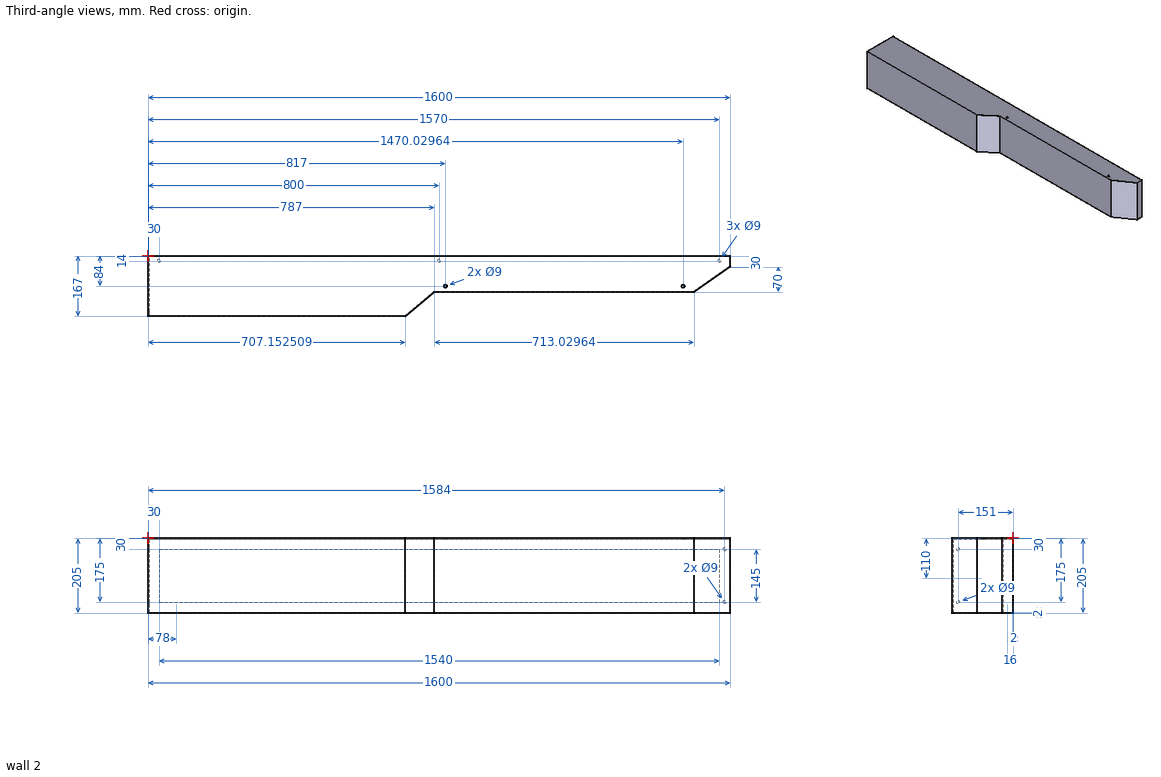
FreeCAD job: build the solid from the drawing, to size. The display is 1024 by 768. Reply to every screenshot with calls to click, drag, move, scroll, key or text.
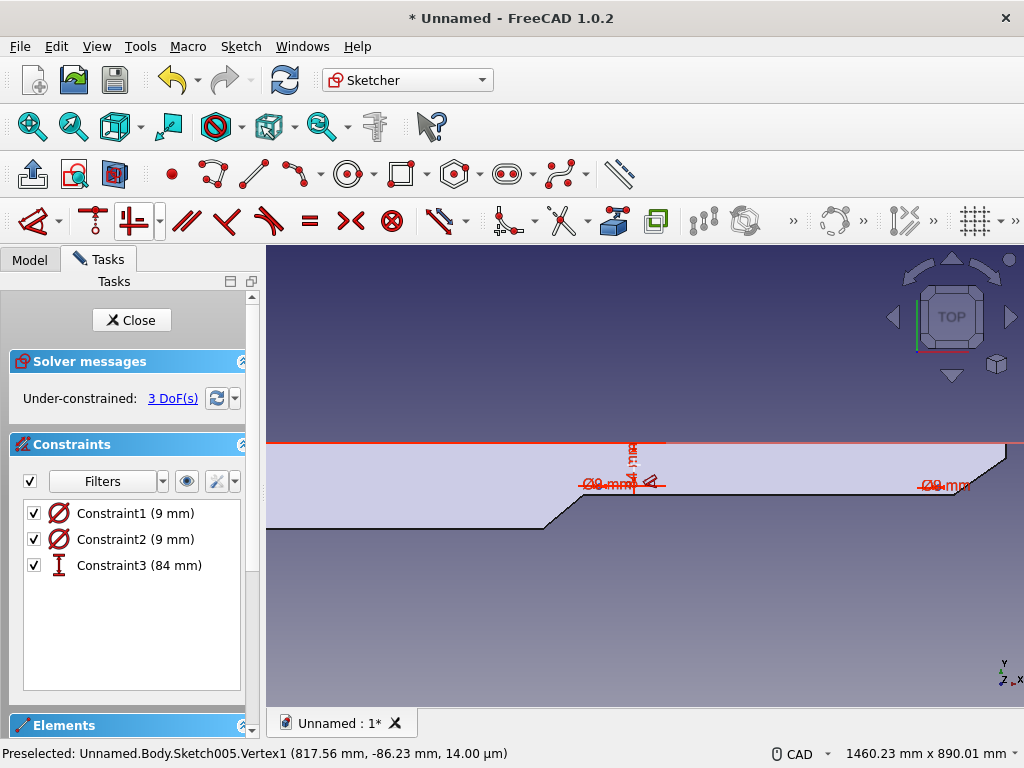
scroll(599, 488, down, 3)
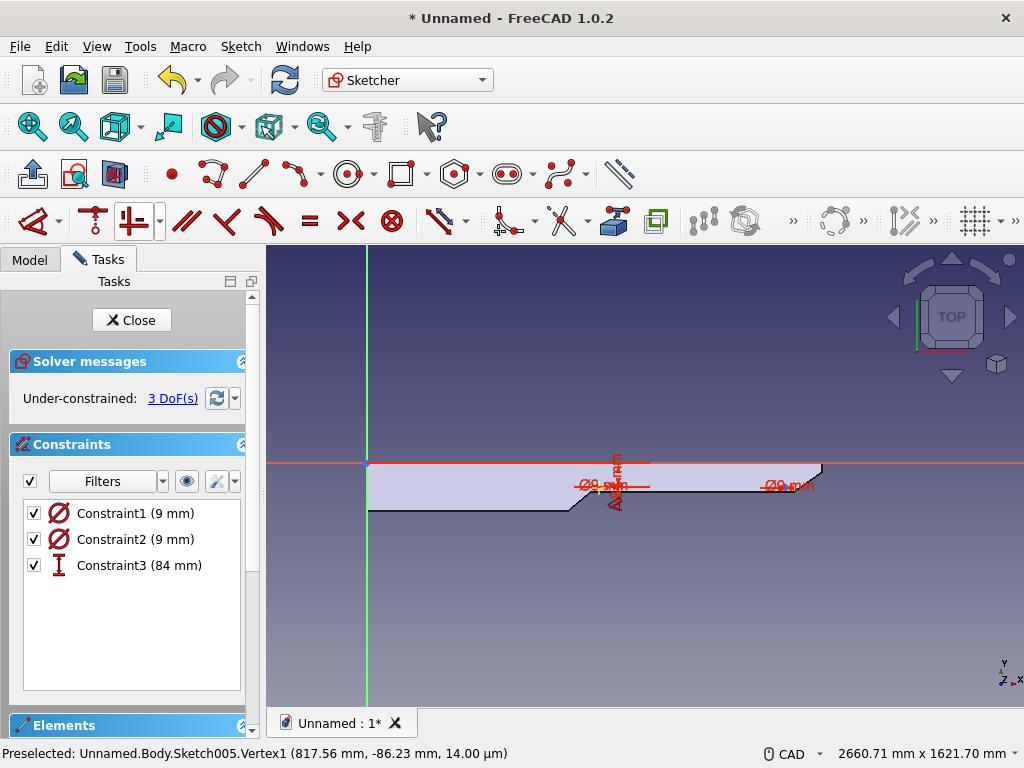
scroll(786, 488, up, 3)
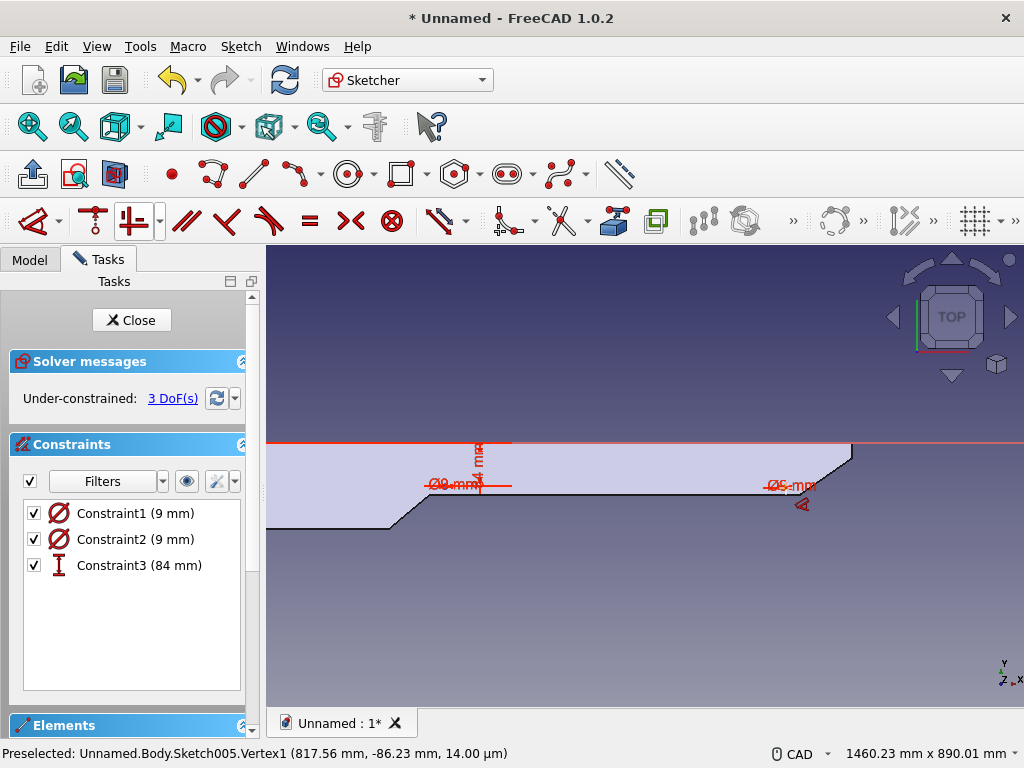
click(785, 488)
click(819, 465)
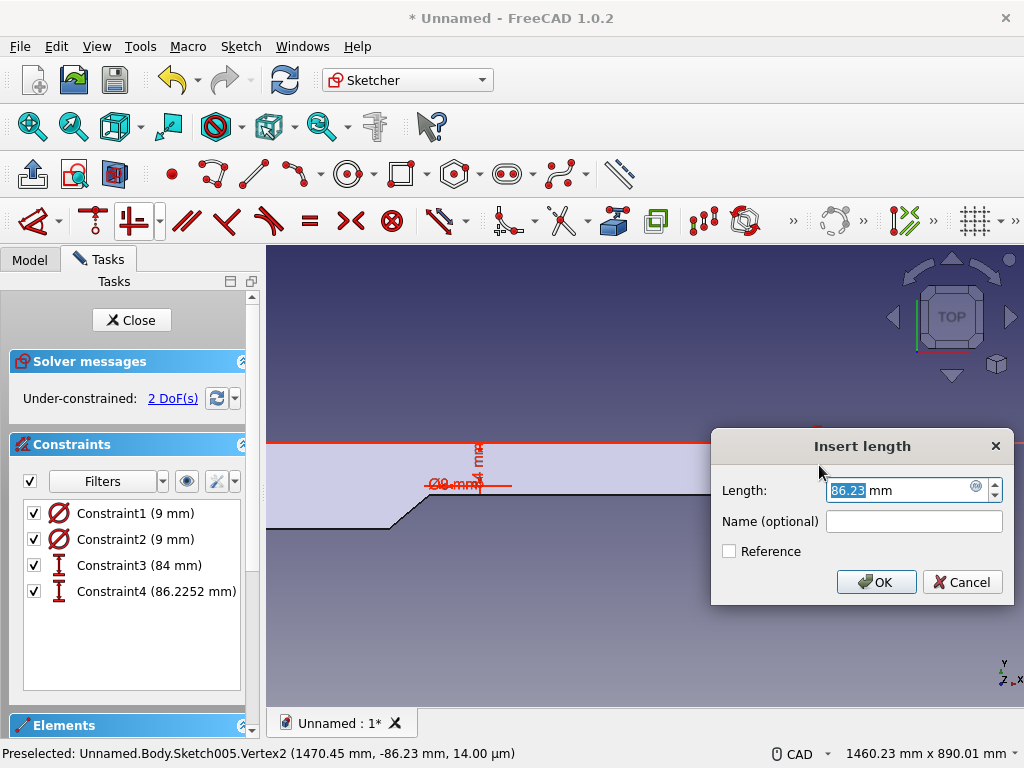
text(84)
key(Return)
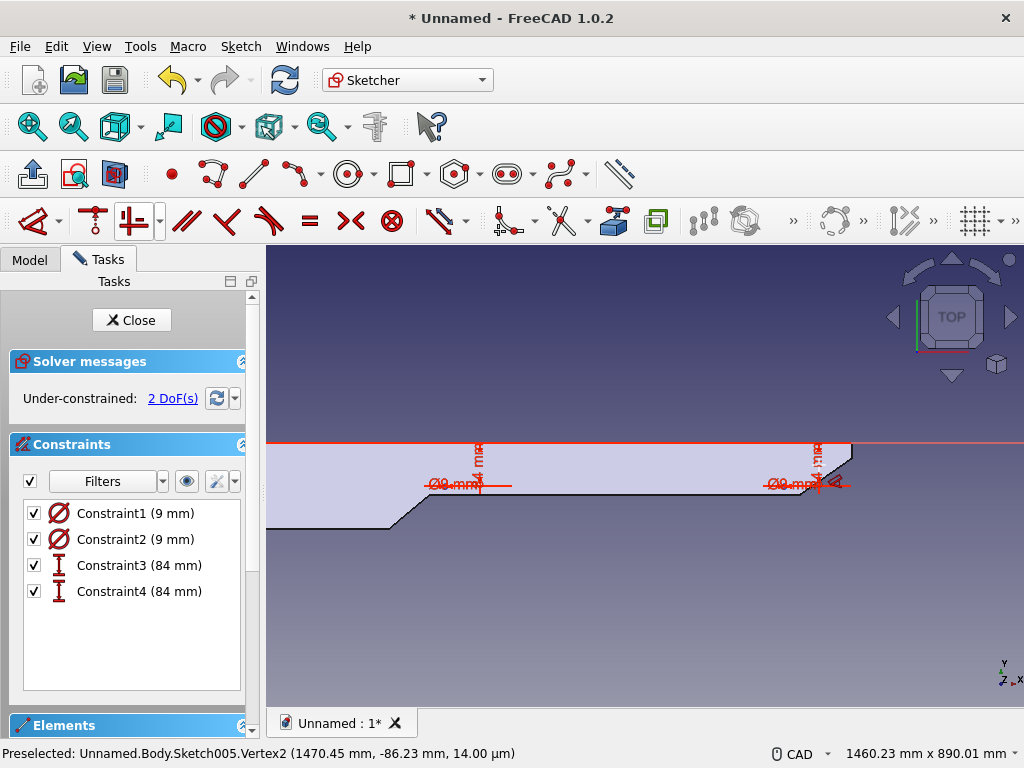
click(446, 486)
click(370, 409)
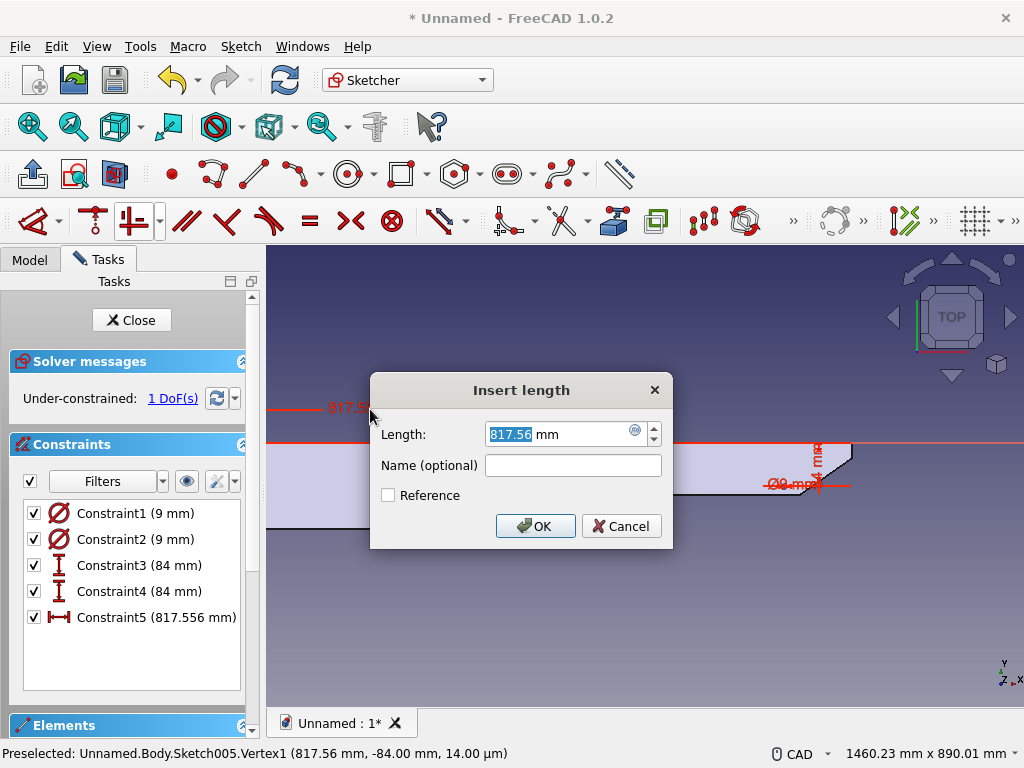
text(817)
key(Return)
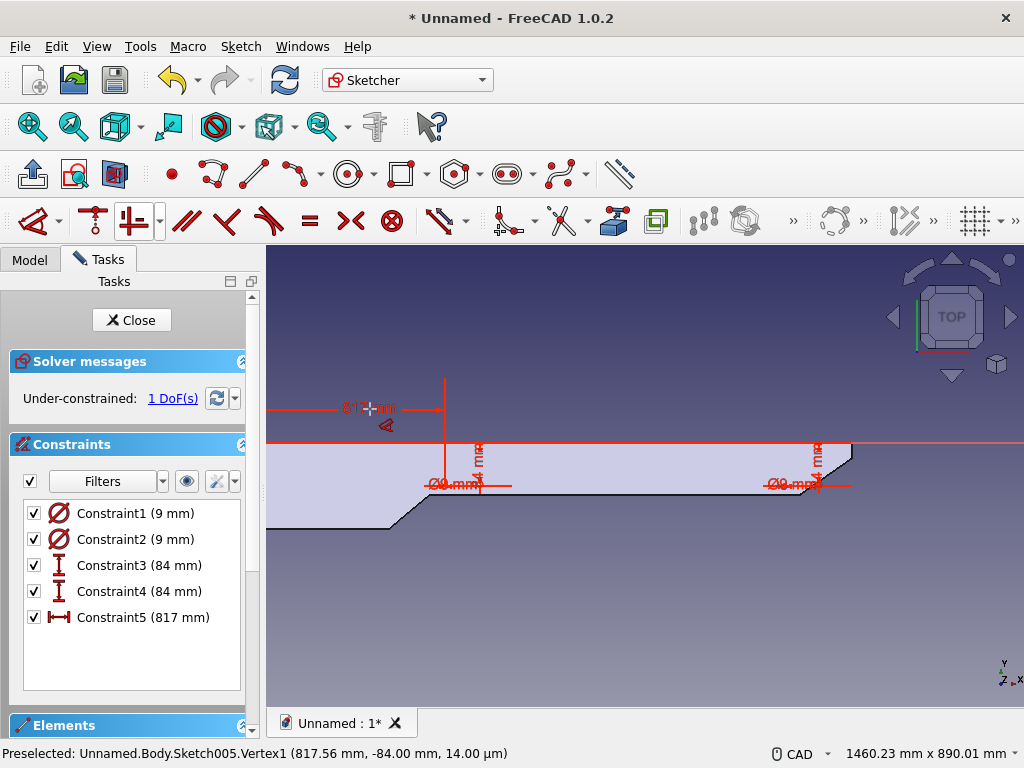
click(785, 486)
click(539, 409)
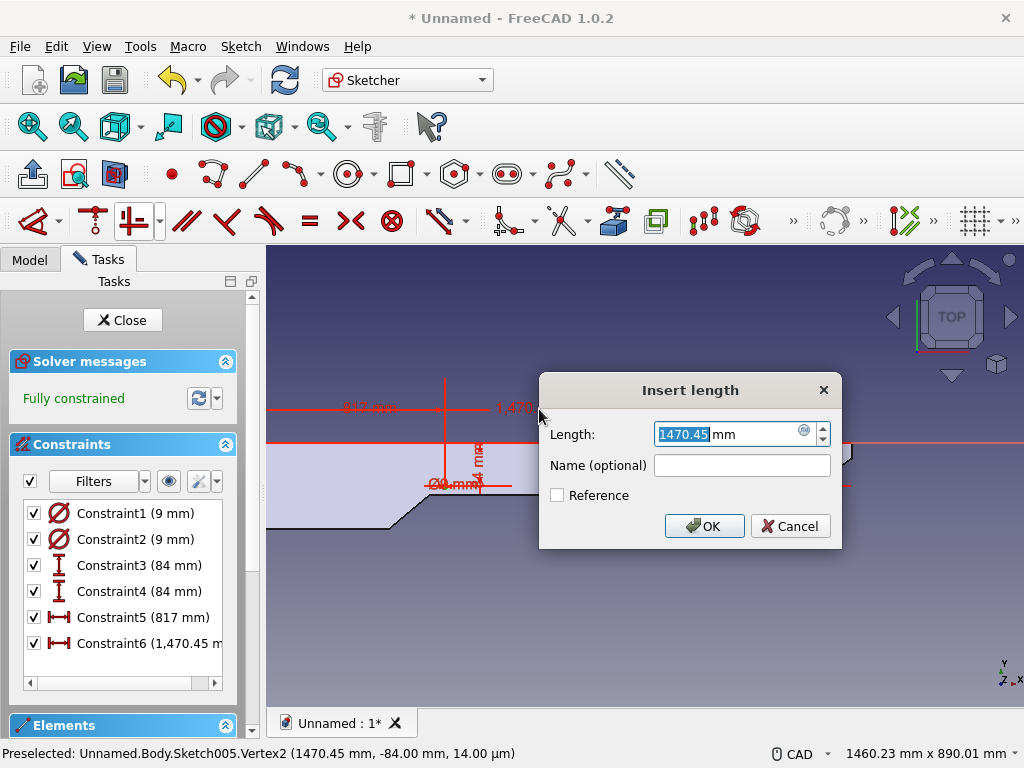
text(1470.02964)
key(Return)
key(Escape)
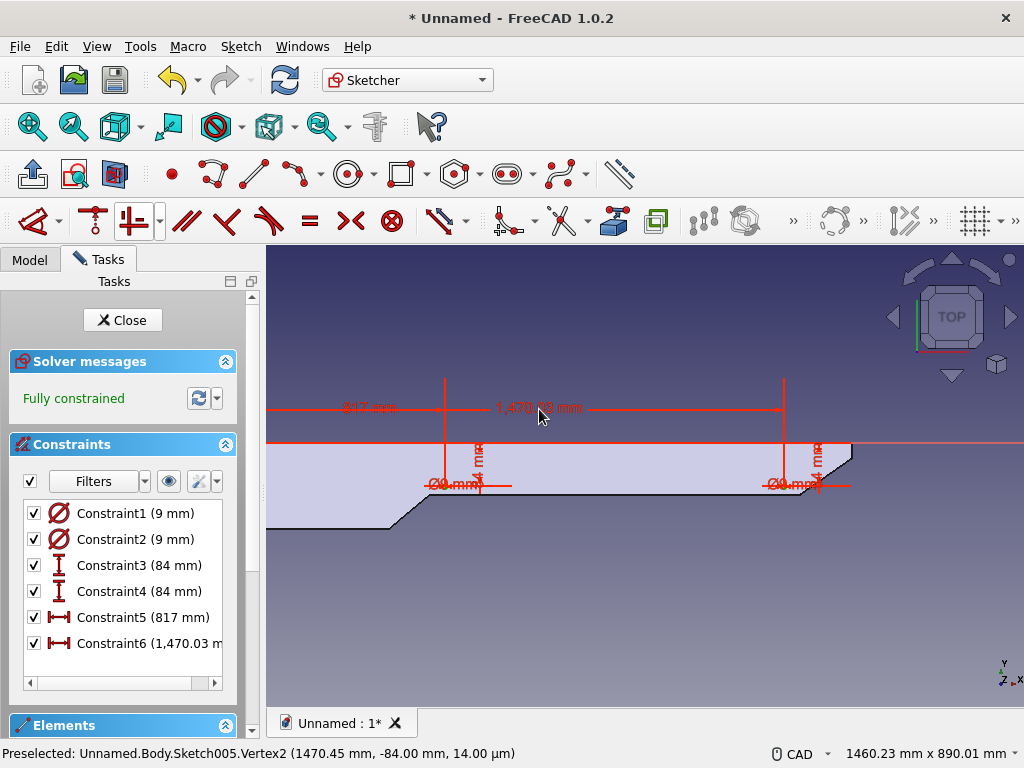
click(123, 320)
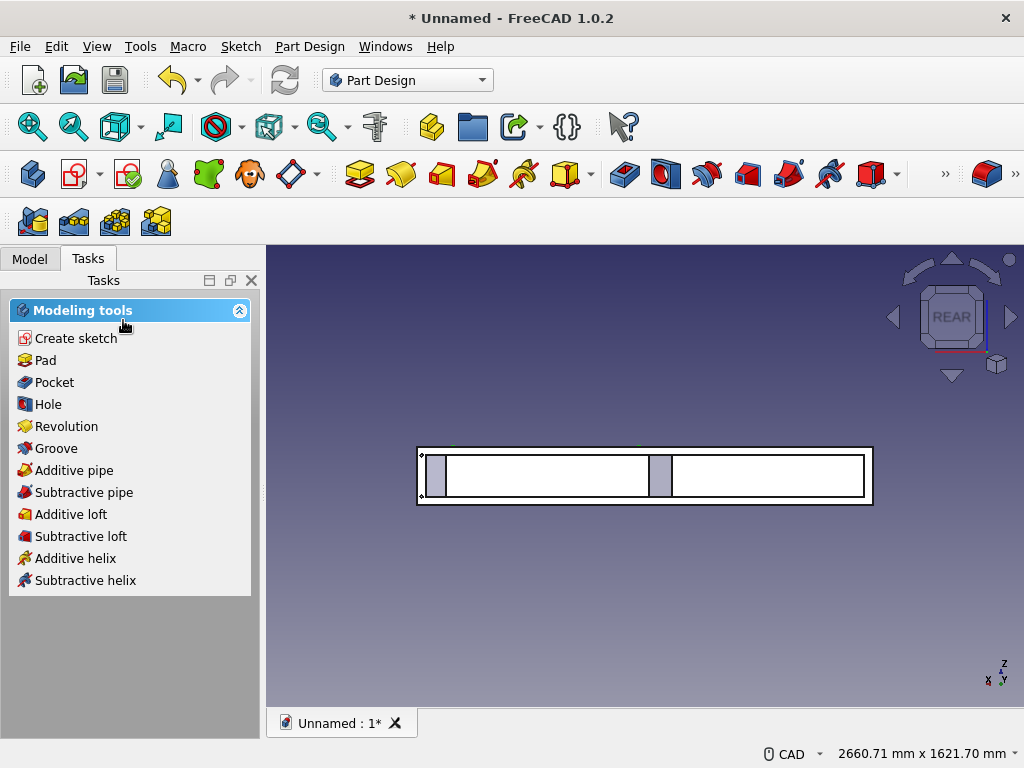
click(625, 174)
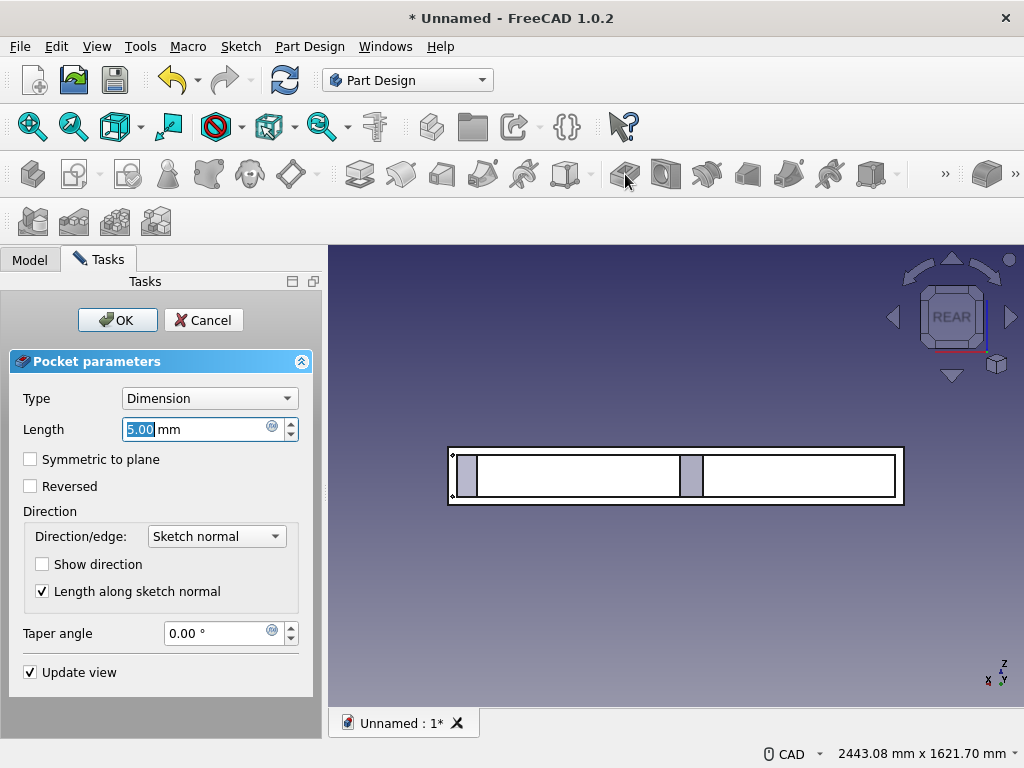
text(110)
key(Tab)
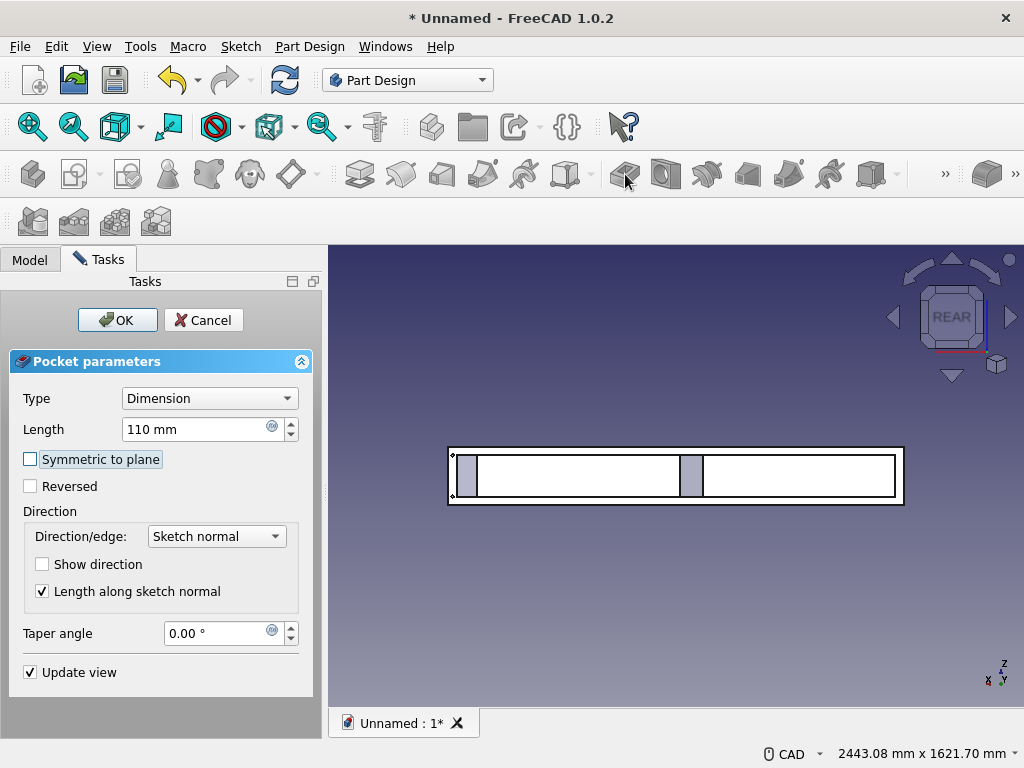
click(118, 320)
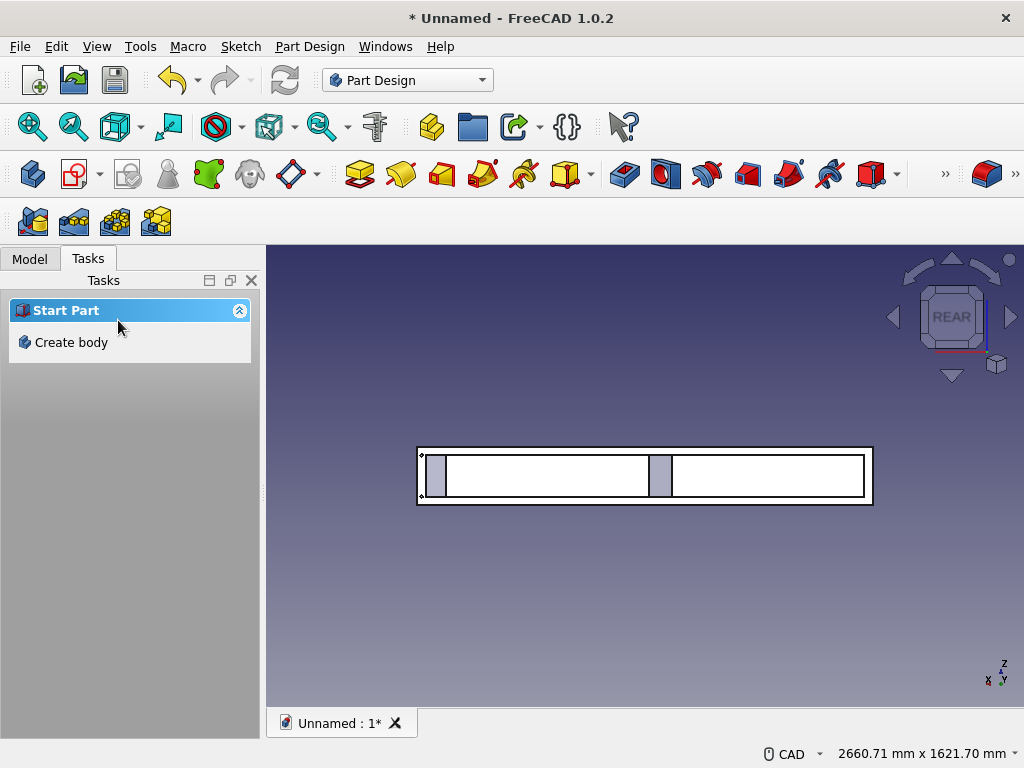
key(0)